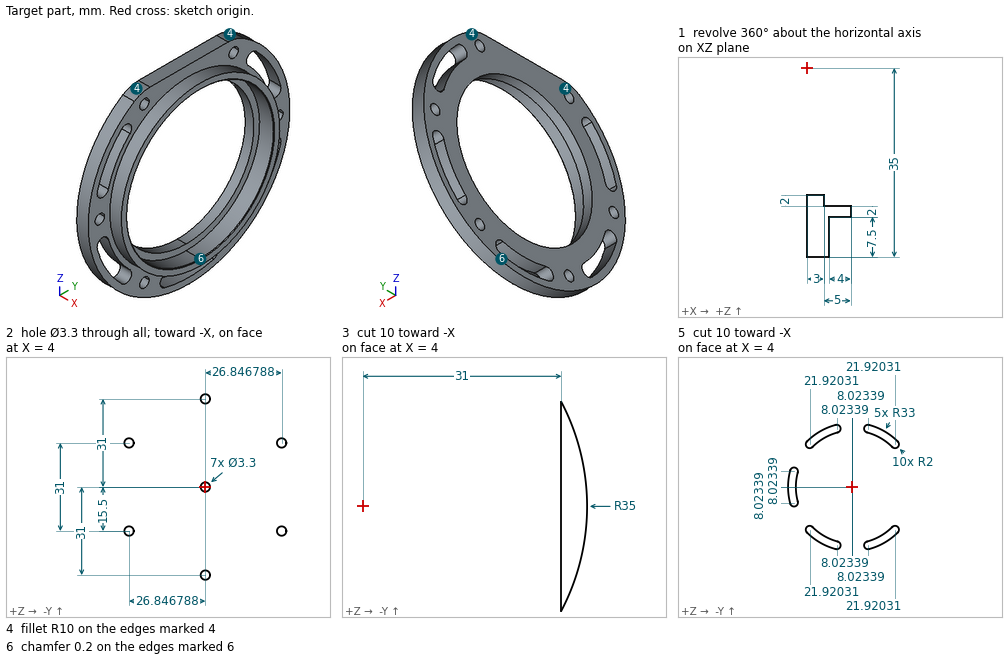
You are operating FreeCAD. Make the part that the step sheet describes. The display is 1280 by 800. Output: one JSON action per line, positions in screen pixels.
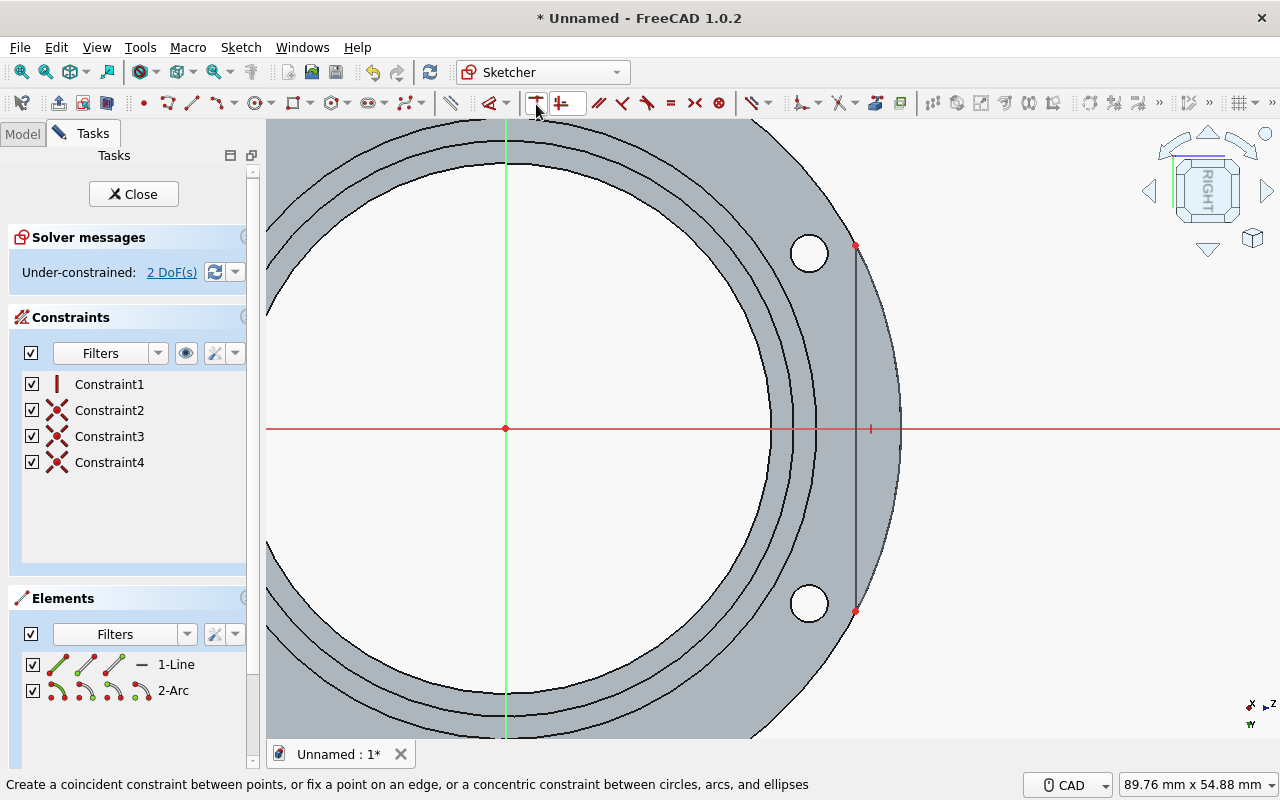
{"action": "left_click", "coordinate": [490, 104]}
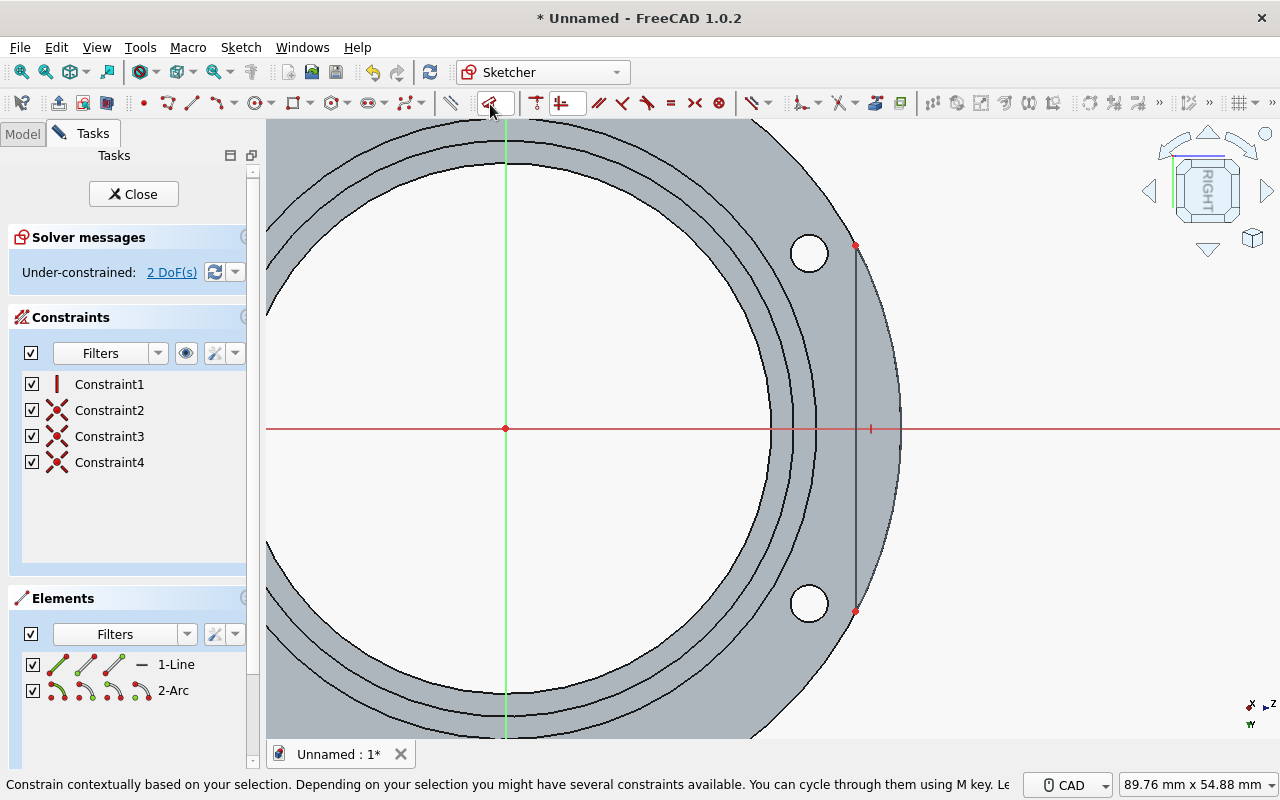
{"action": "left_click", "coordinate": [894, 504]}
{"action": "left_click", "coordinate": [925, 510]}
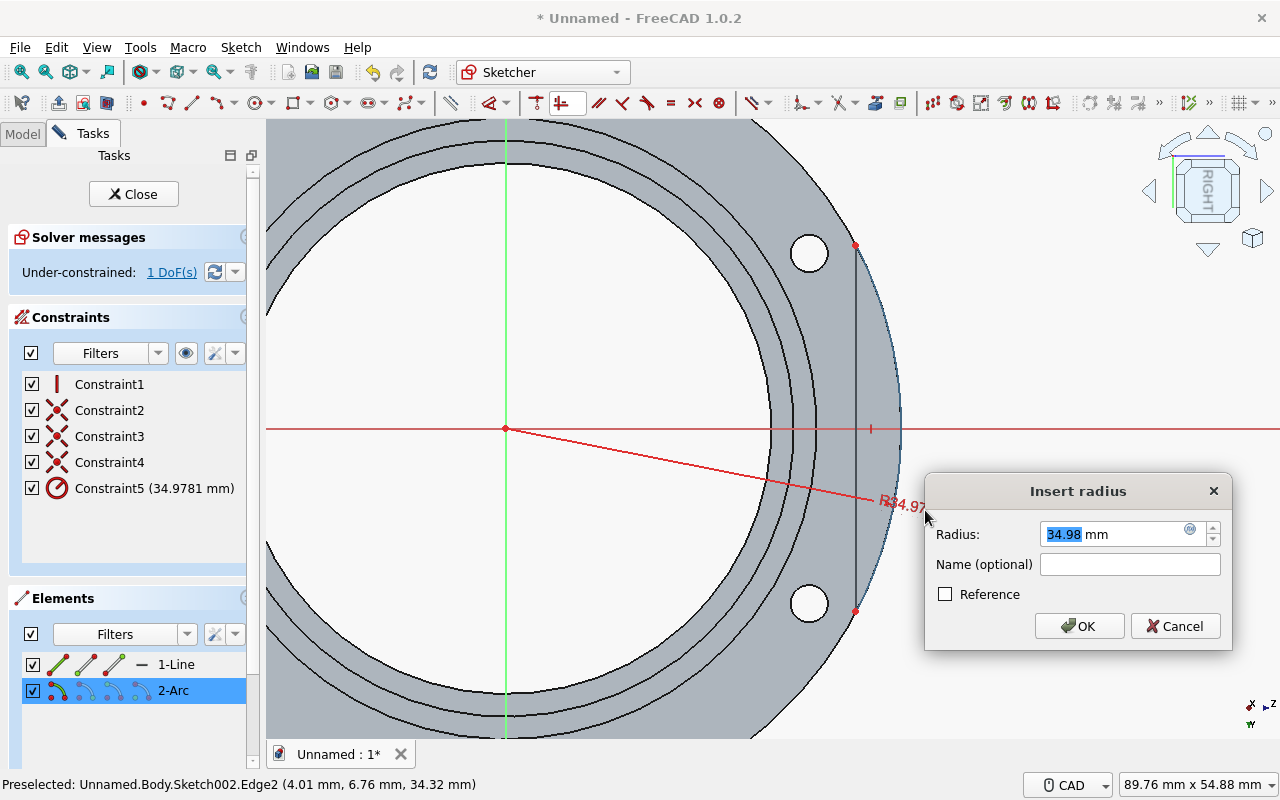
{"action": "type", "text": "35"}
{"action": "key", "text": "Return"}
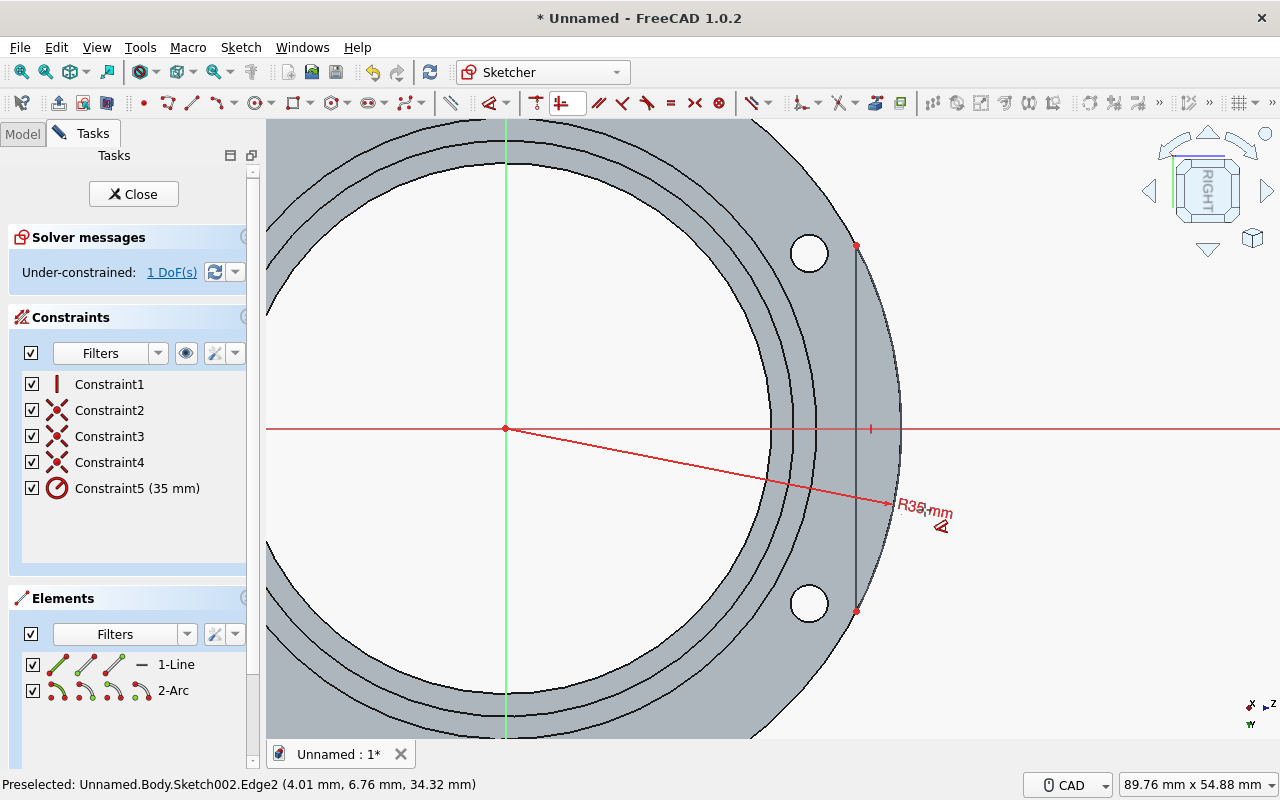
{"action": "left_click", "coordinate": [856, 245]}
{"action": "left_click", "coordinate": [681, 211]}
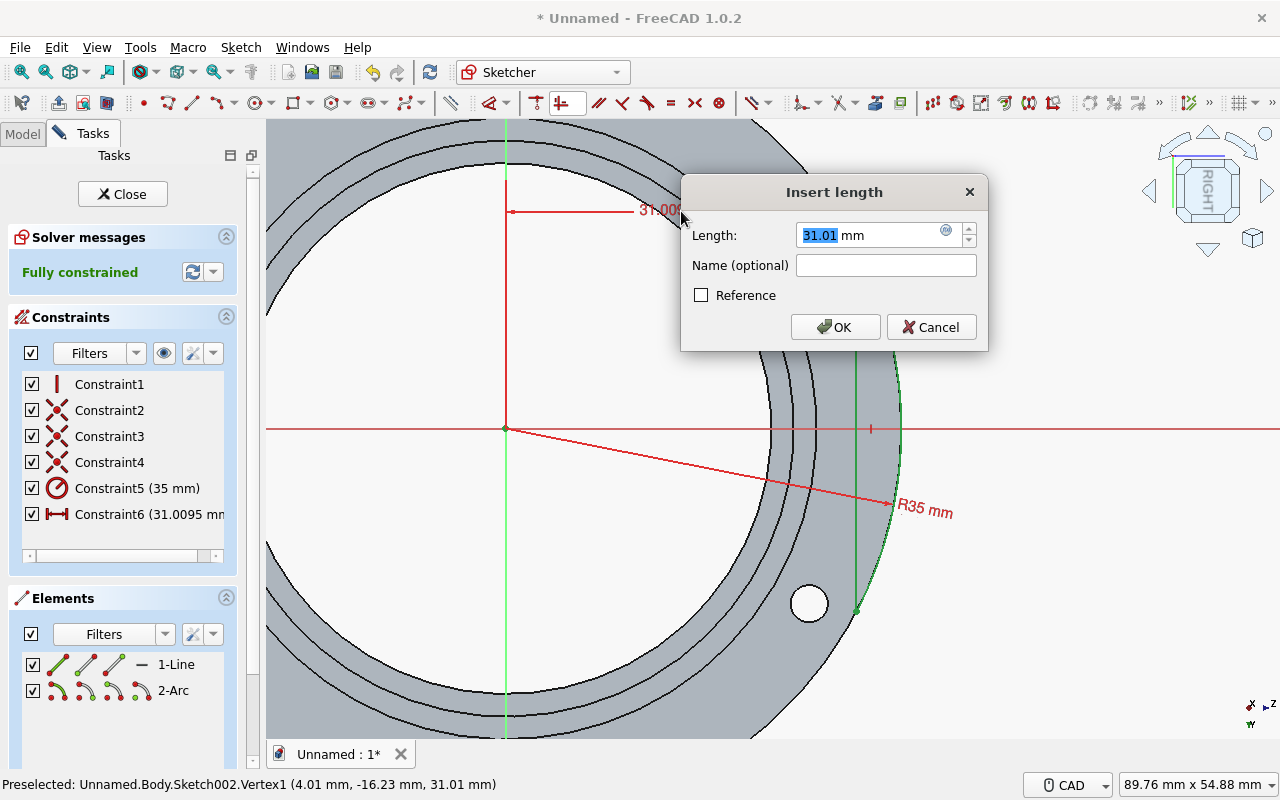
{"action": "type", "text": "31"}
{"action": "key", "text": "Return"}
{"action": "key", "text": "Escape"}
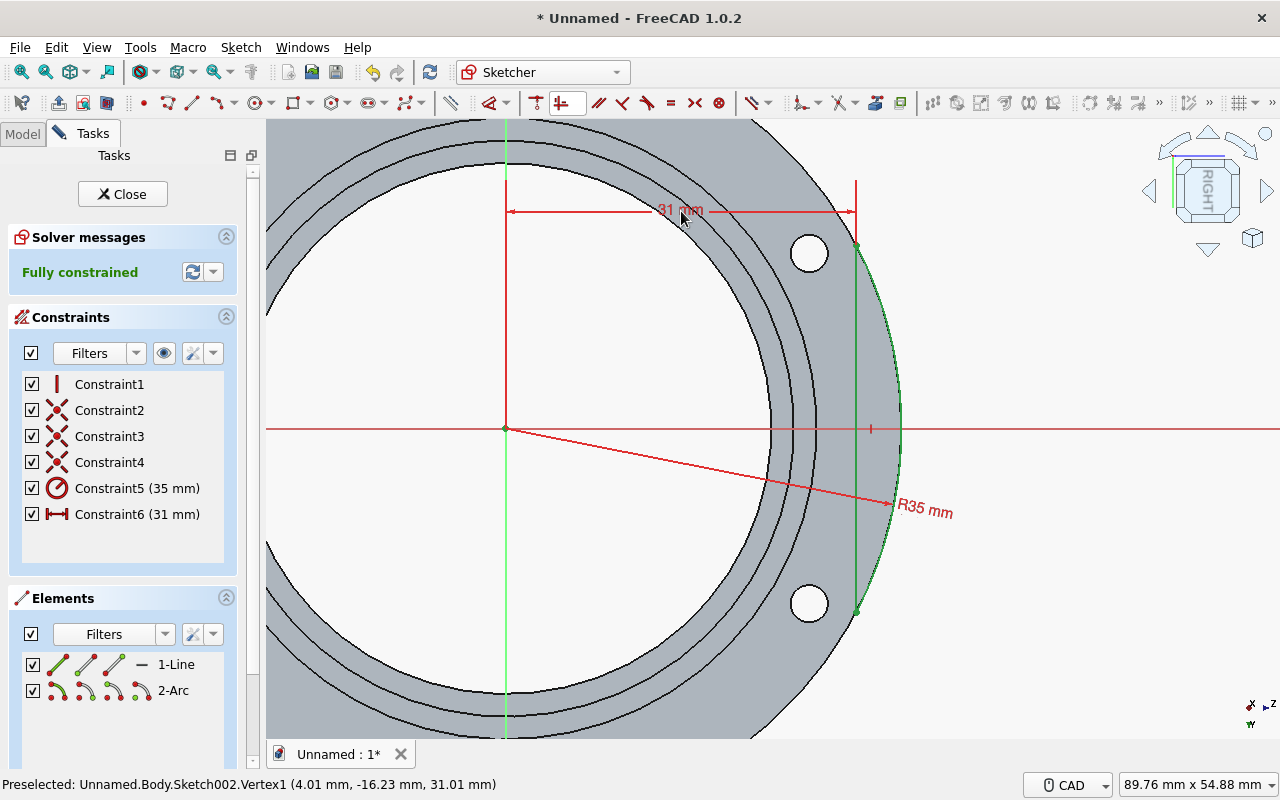
{"action": "left_click", "coordinate": [123, 194]}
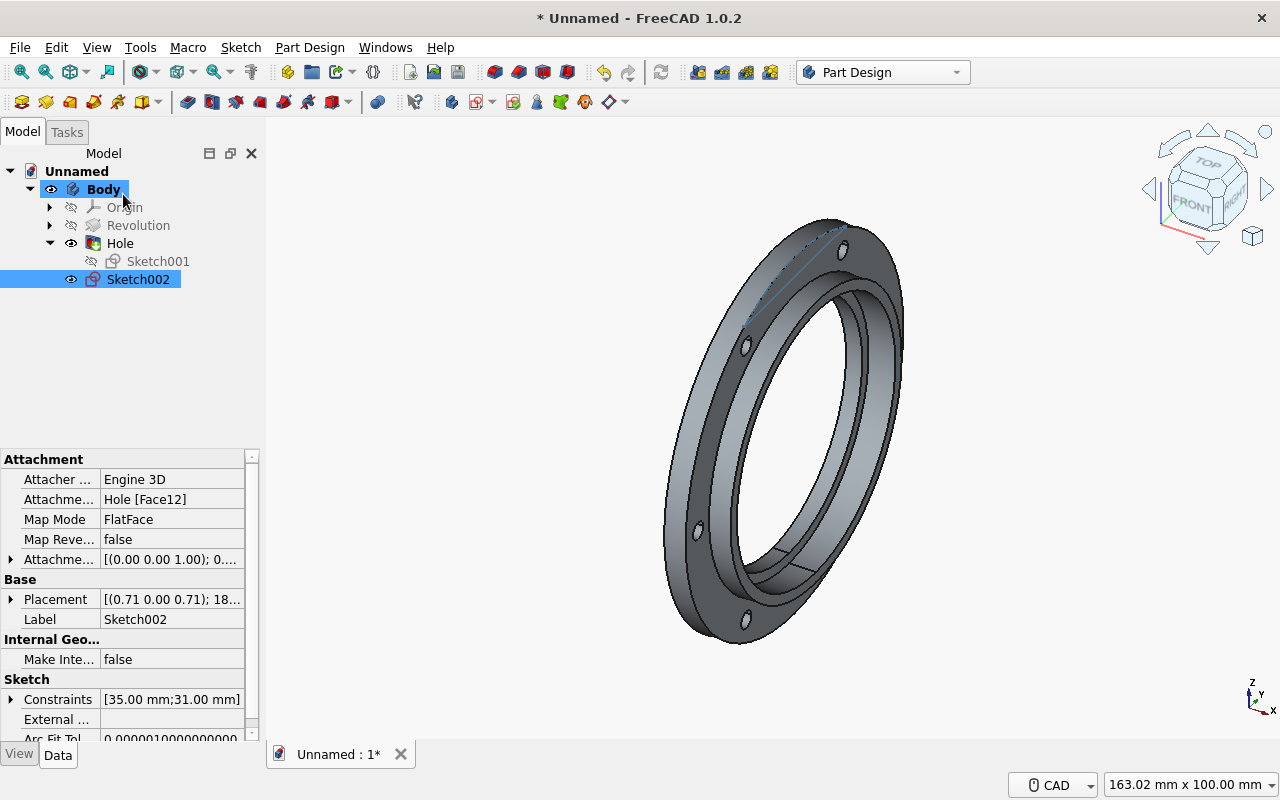
{"action": "left_click", "coordinate": [188, 102]}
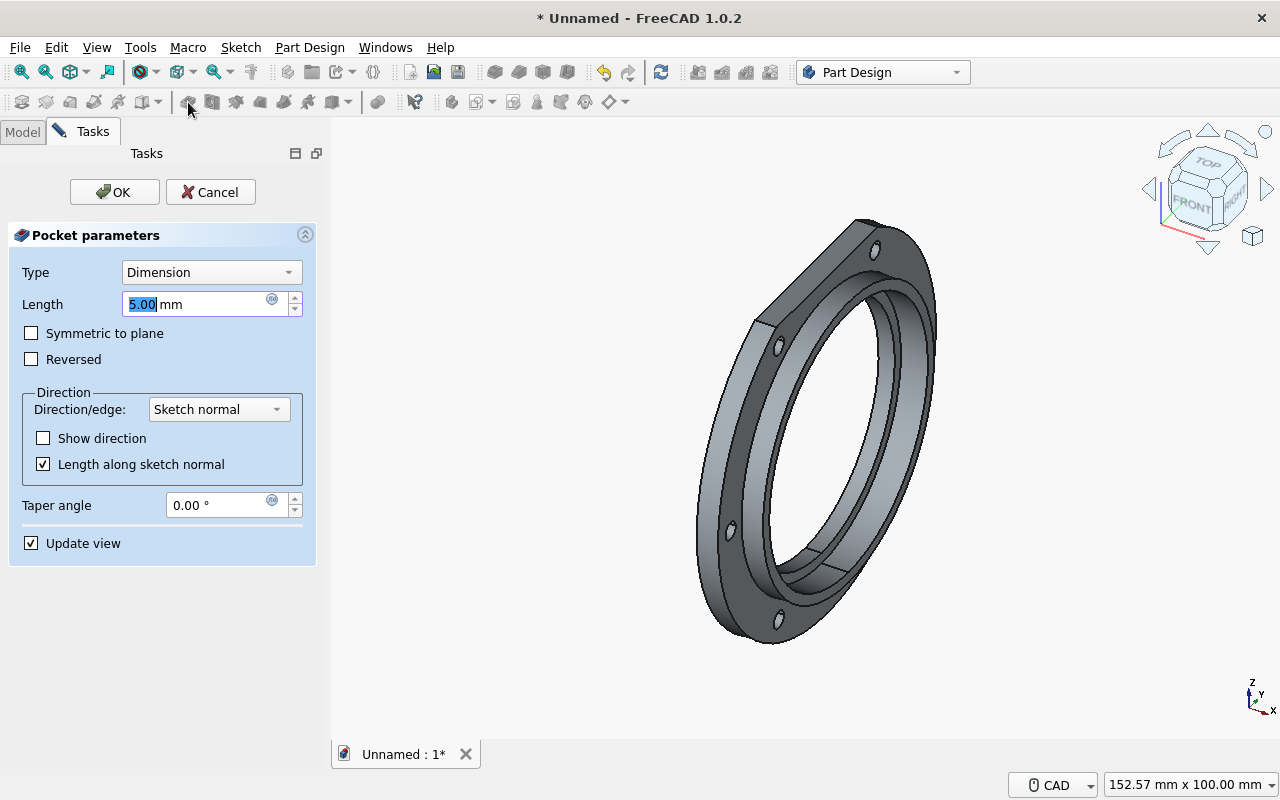
{"action": "type", "text": "10"}
{"action": "key", "text": "Tab"}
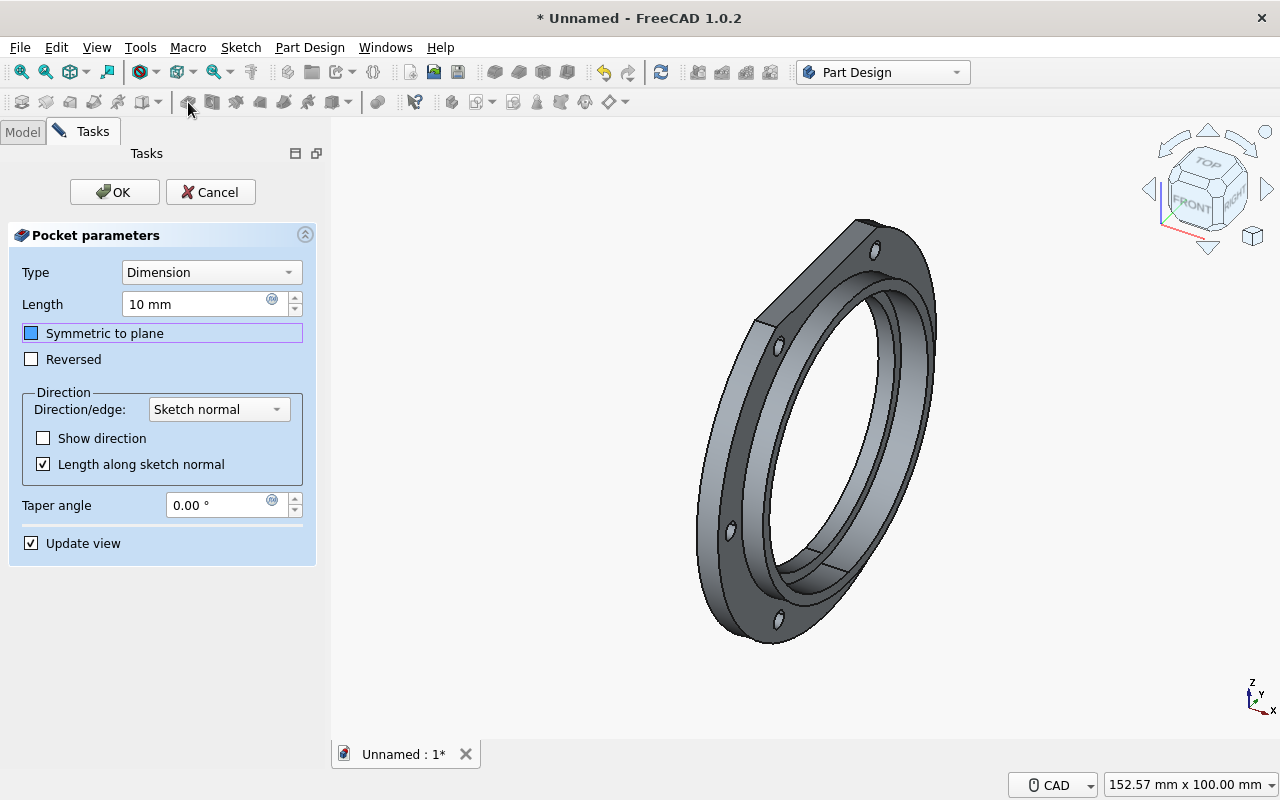
{"action": "left_click", "coordinate": [115, 192]}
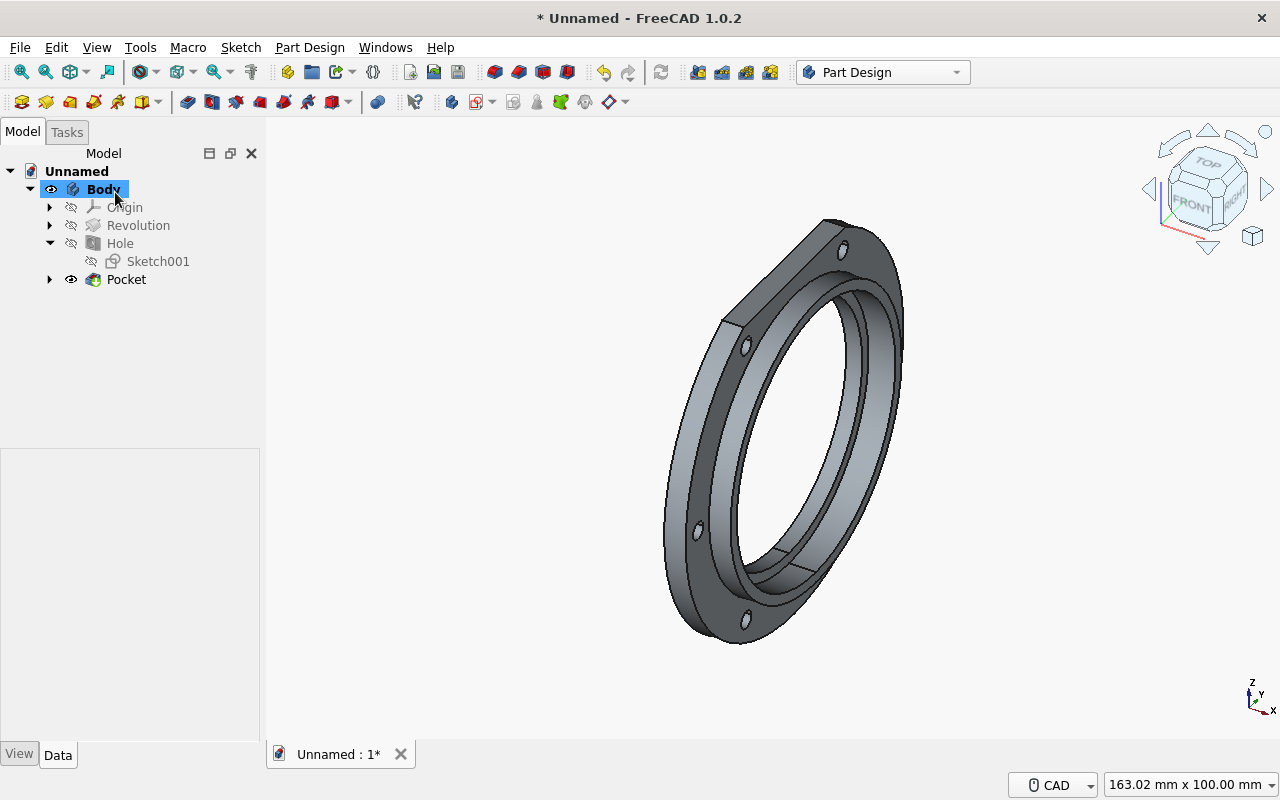
{"action": "key", "text": "0"}